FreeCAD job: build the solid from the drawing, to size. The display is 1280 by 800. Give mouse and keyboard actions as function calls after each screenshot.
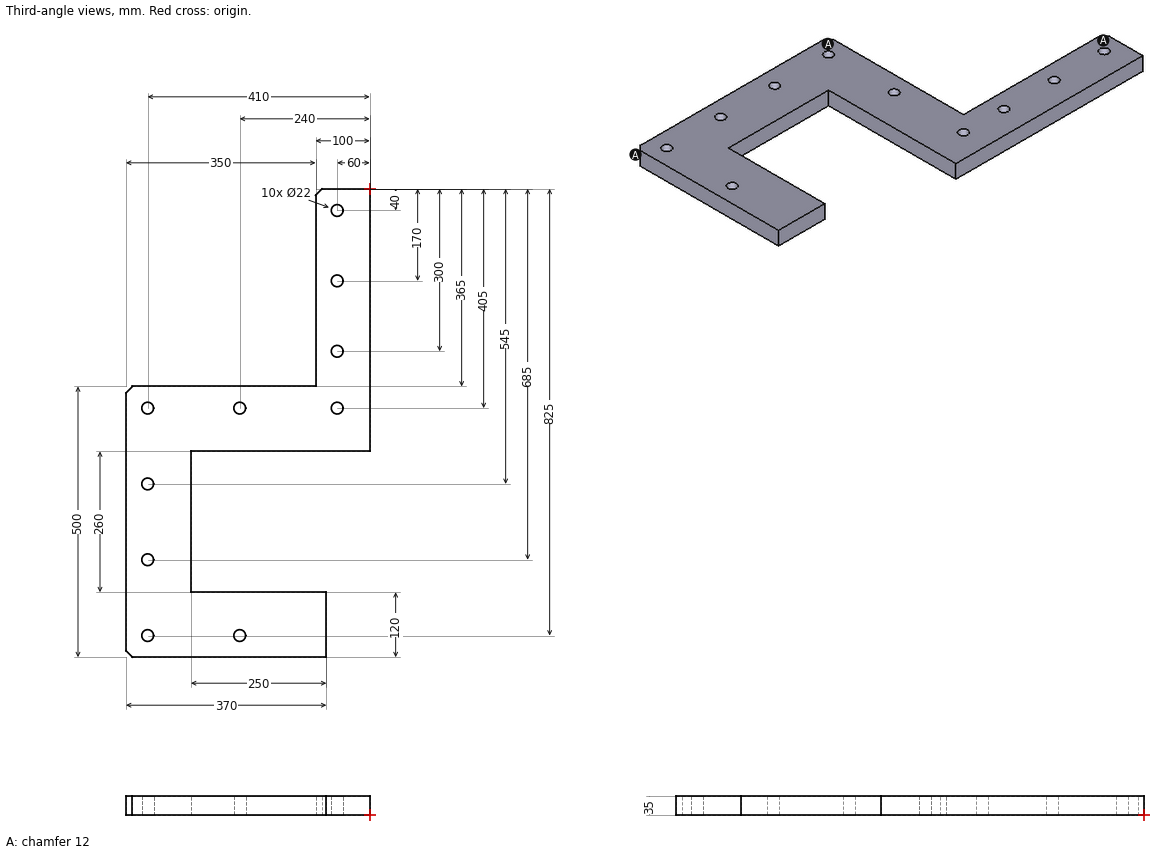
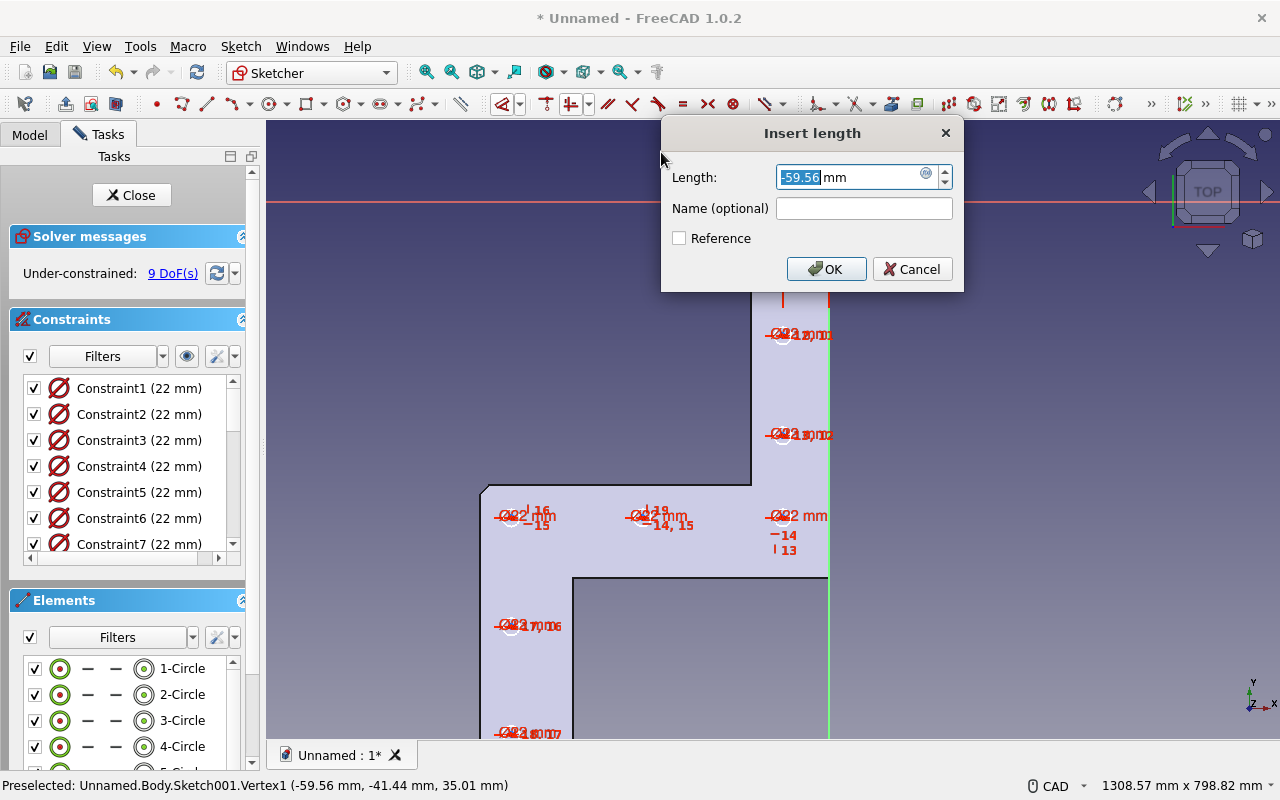
text(-60)
key(Return)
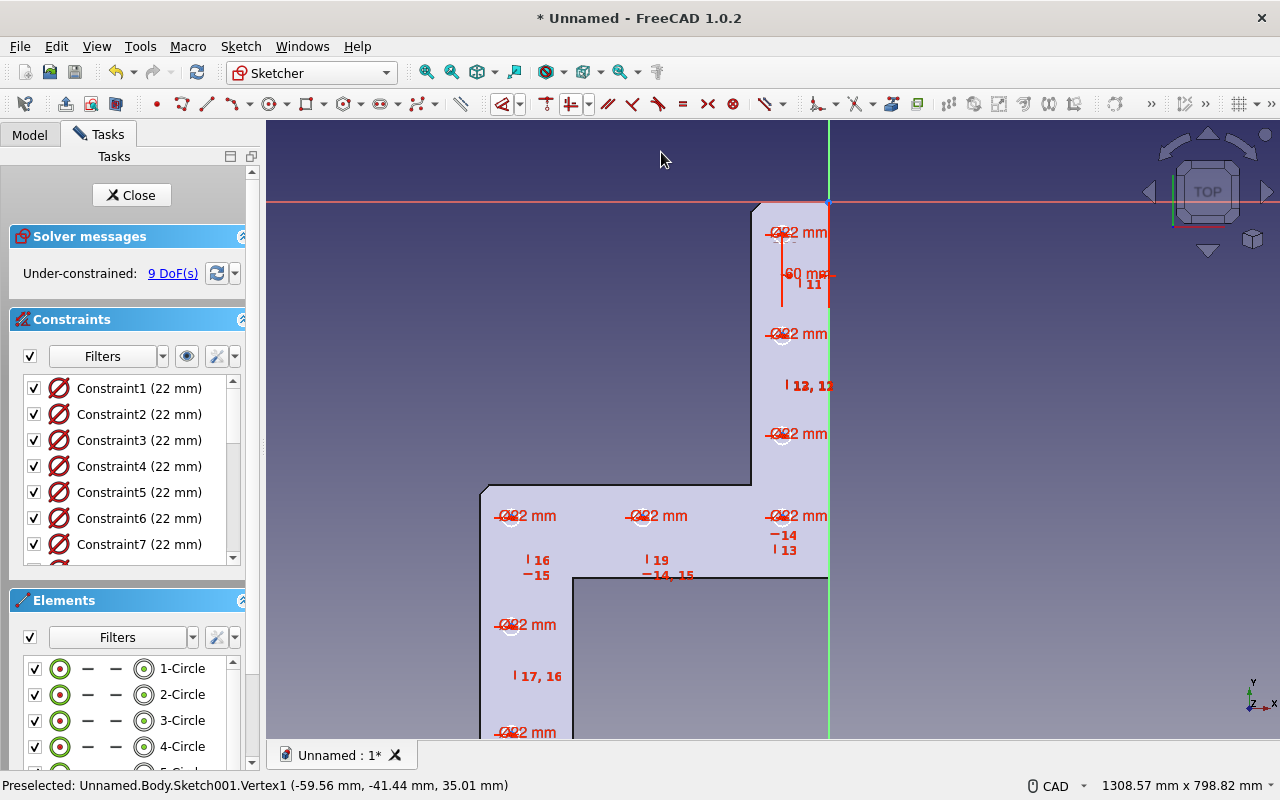
scroll(782, 235, up, 2)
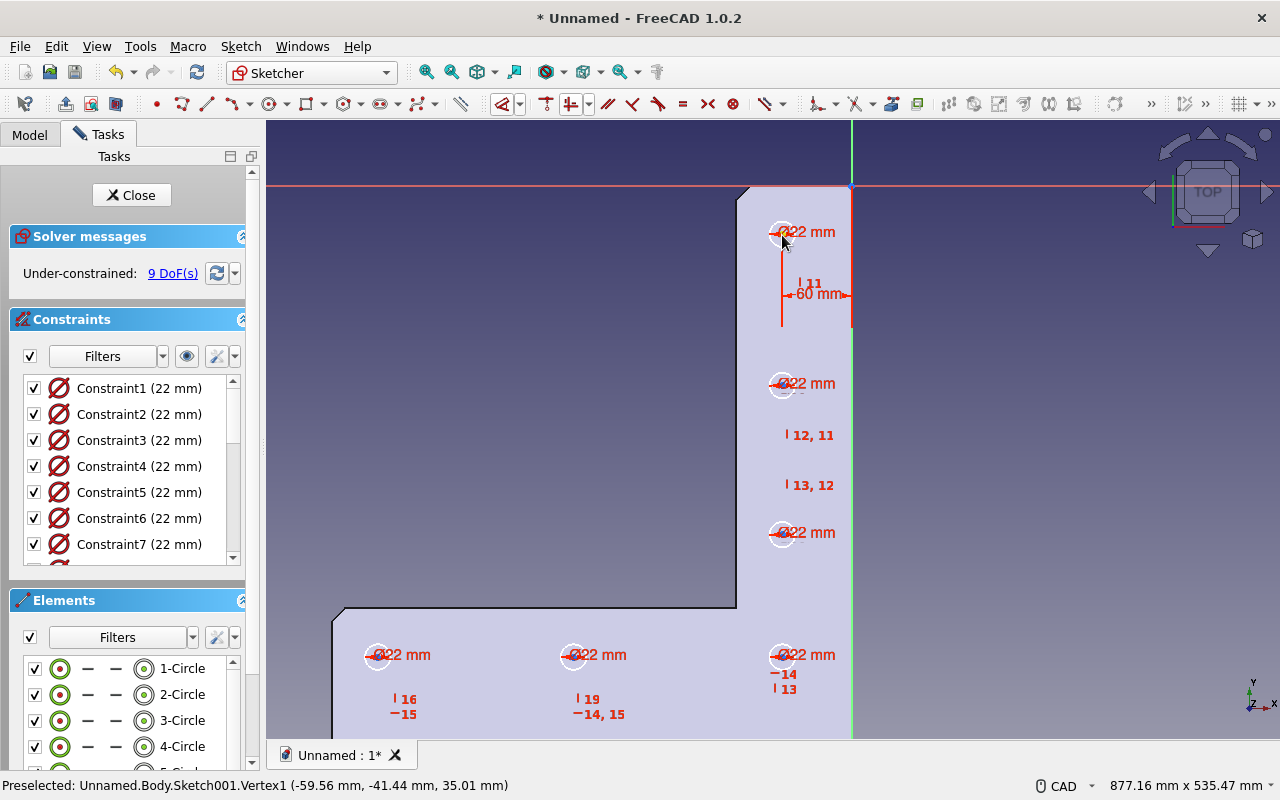
click(782, 234)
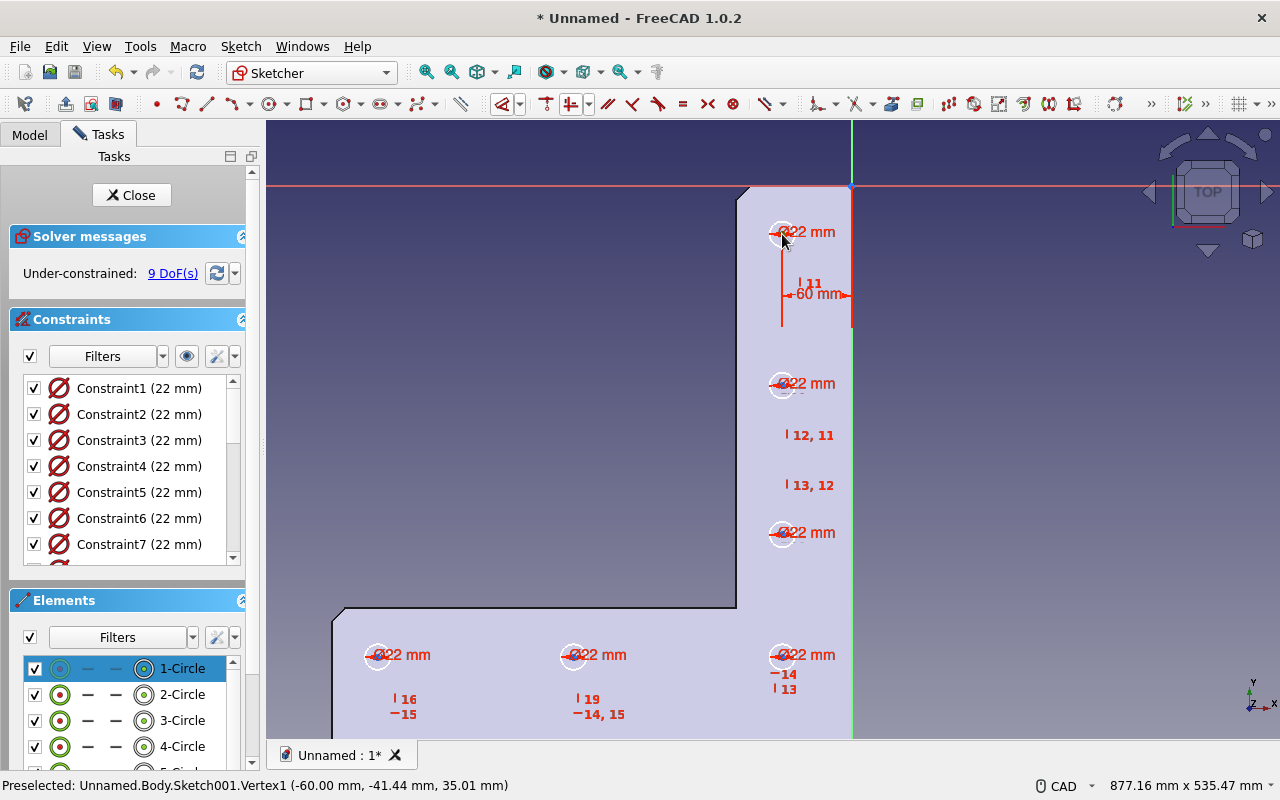
click(520, 104)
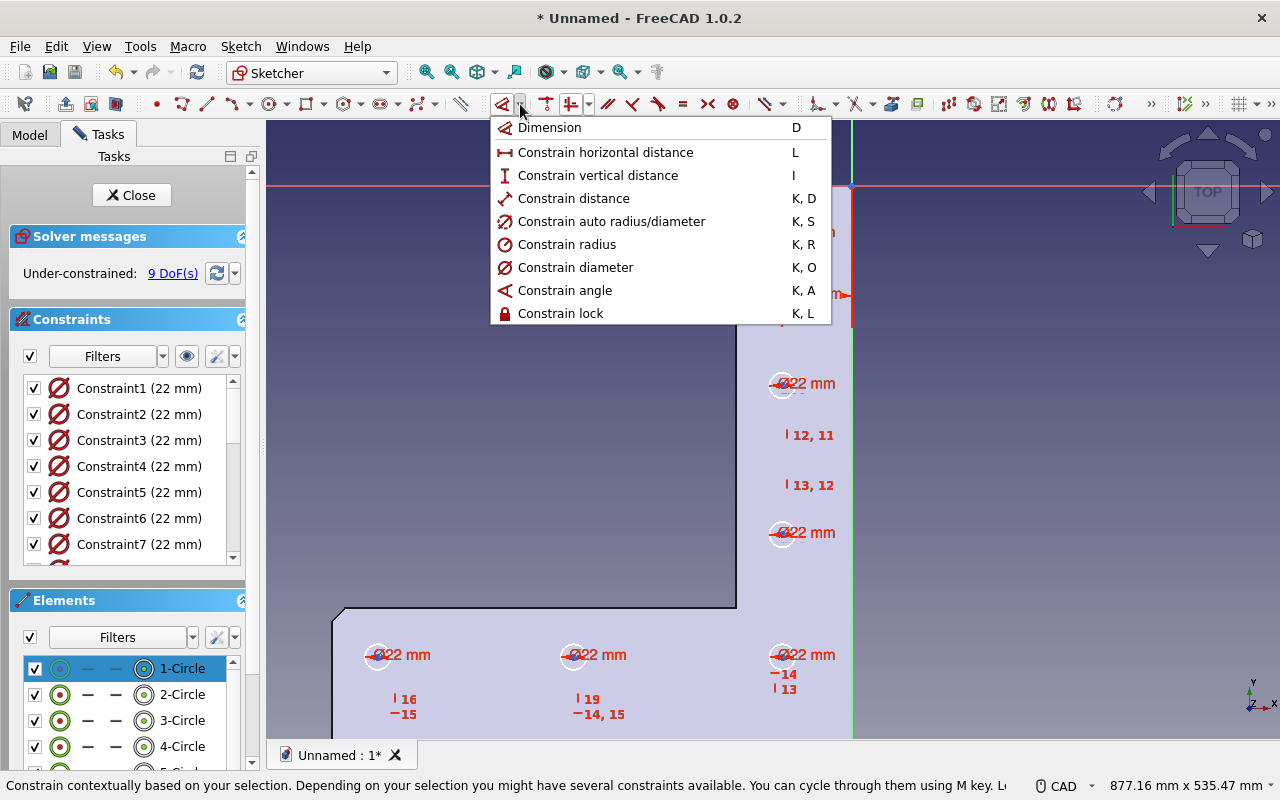
click(661, 176)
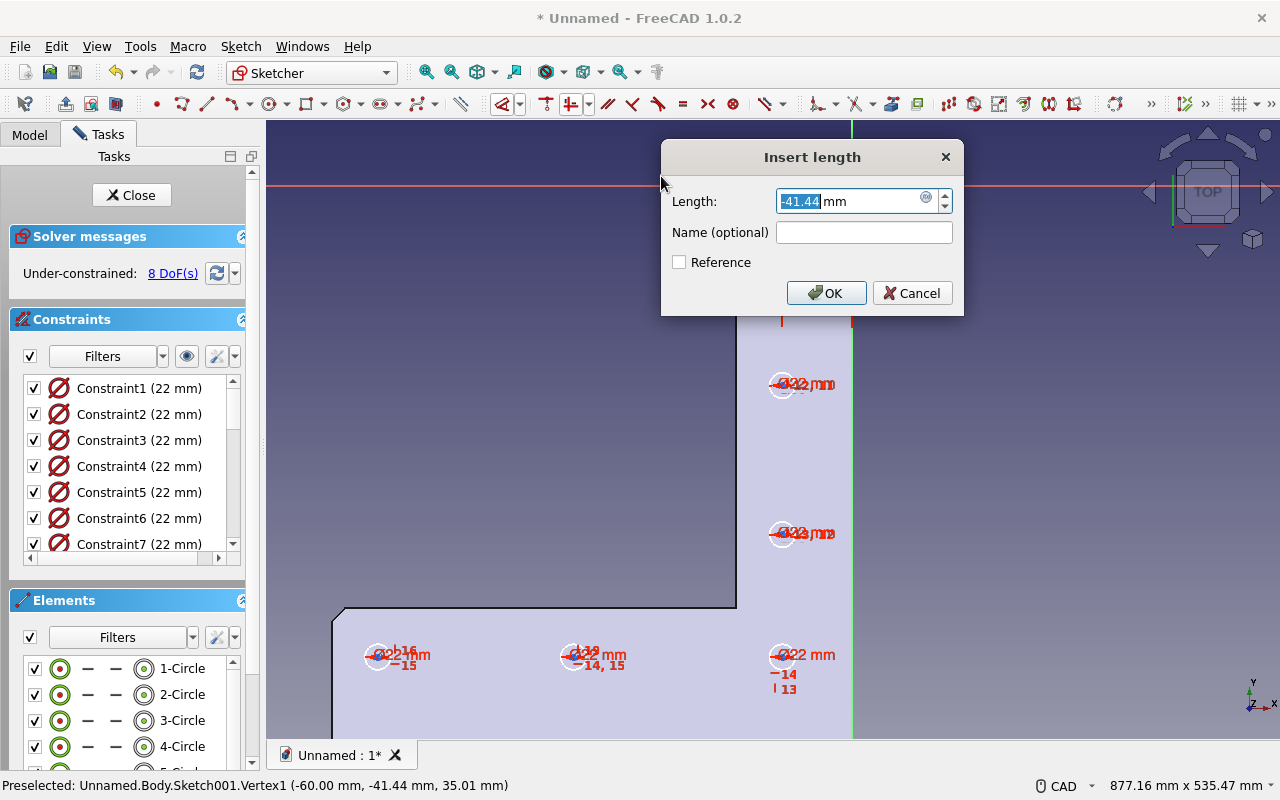
text(-40)
key(Return)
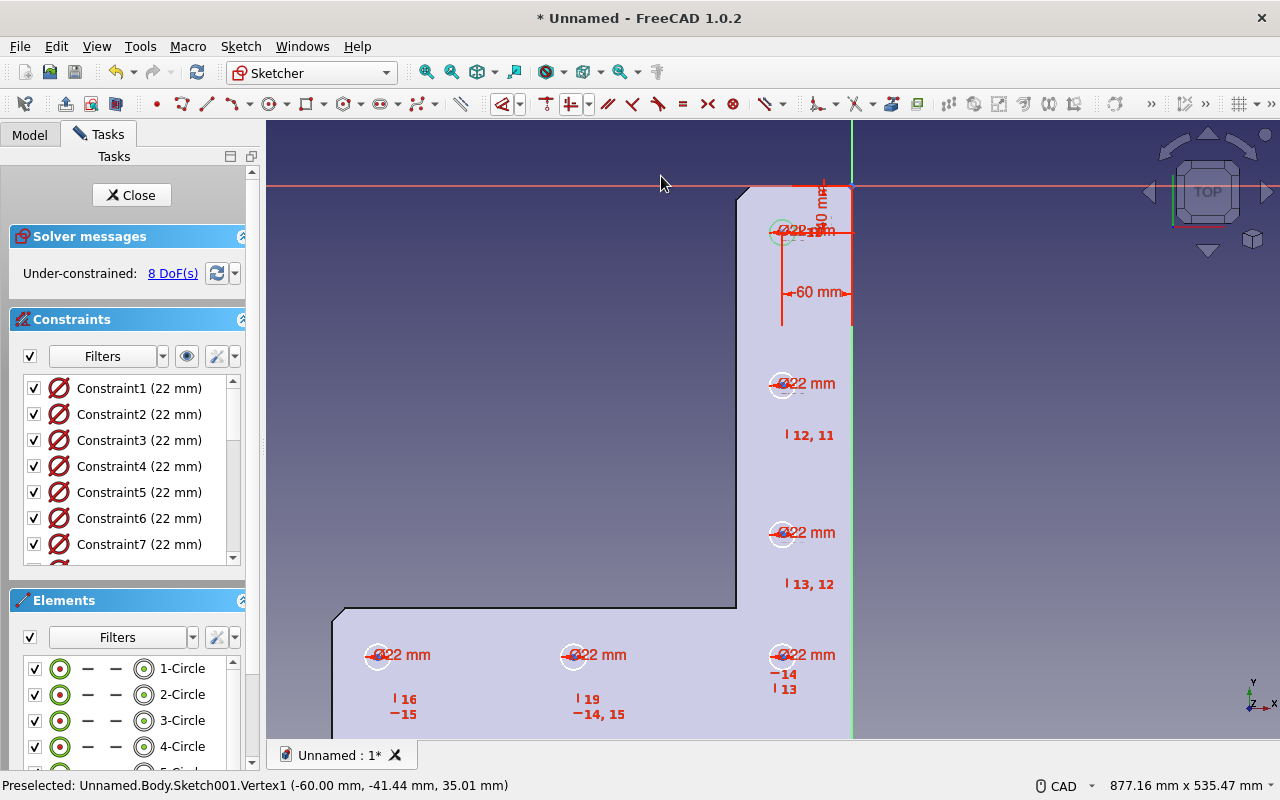
click(782, 386)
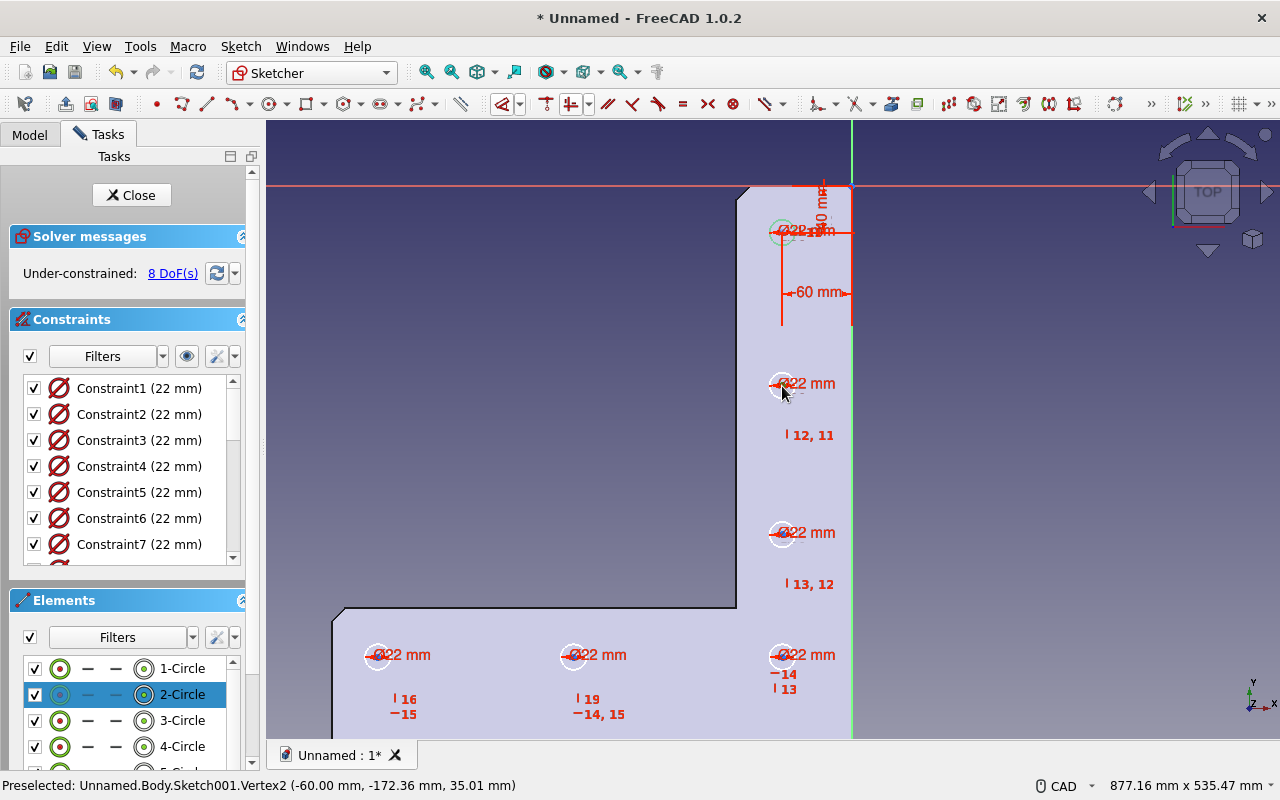
click(520, 104)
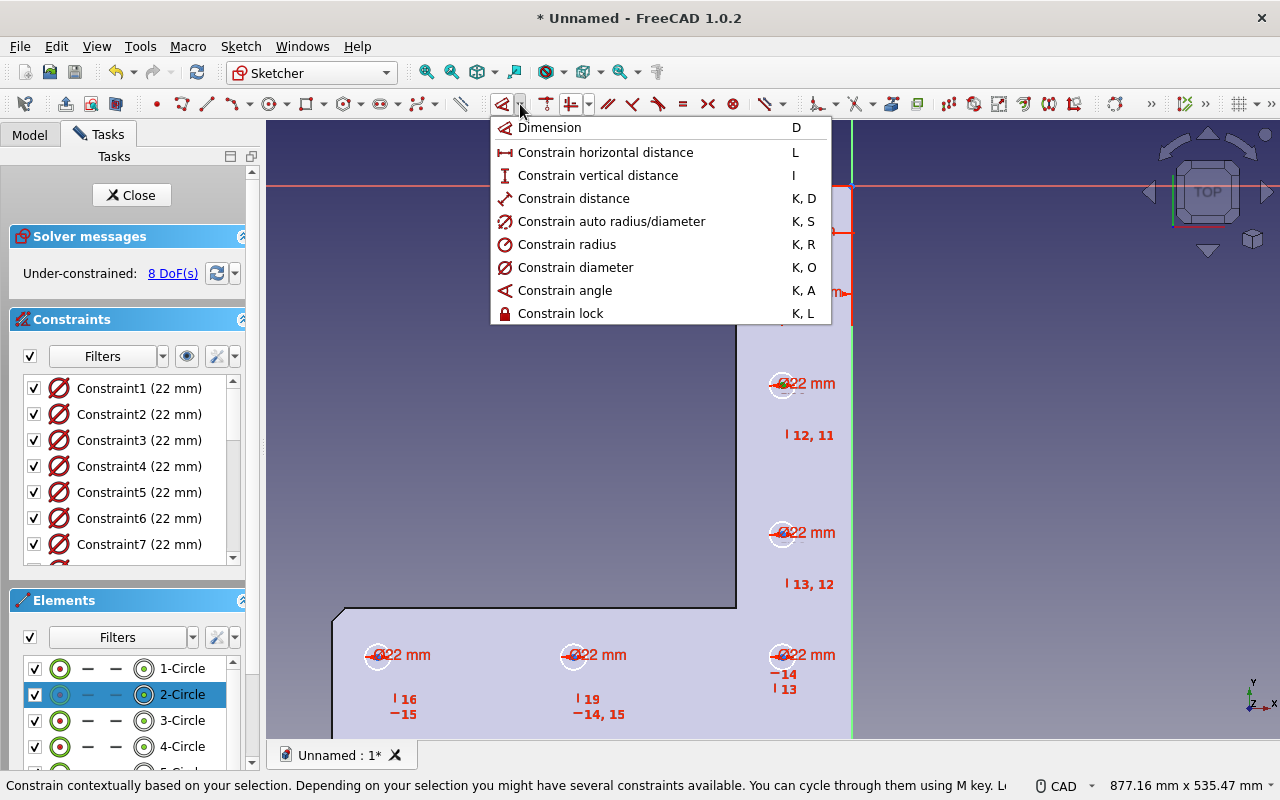
click(661, 176)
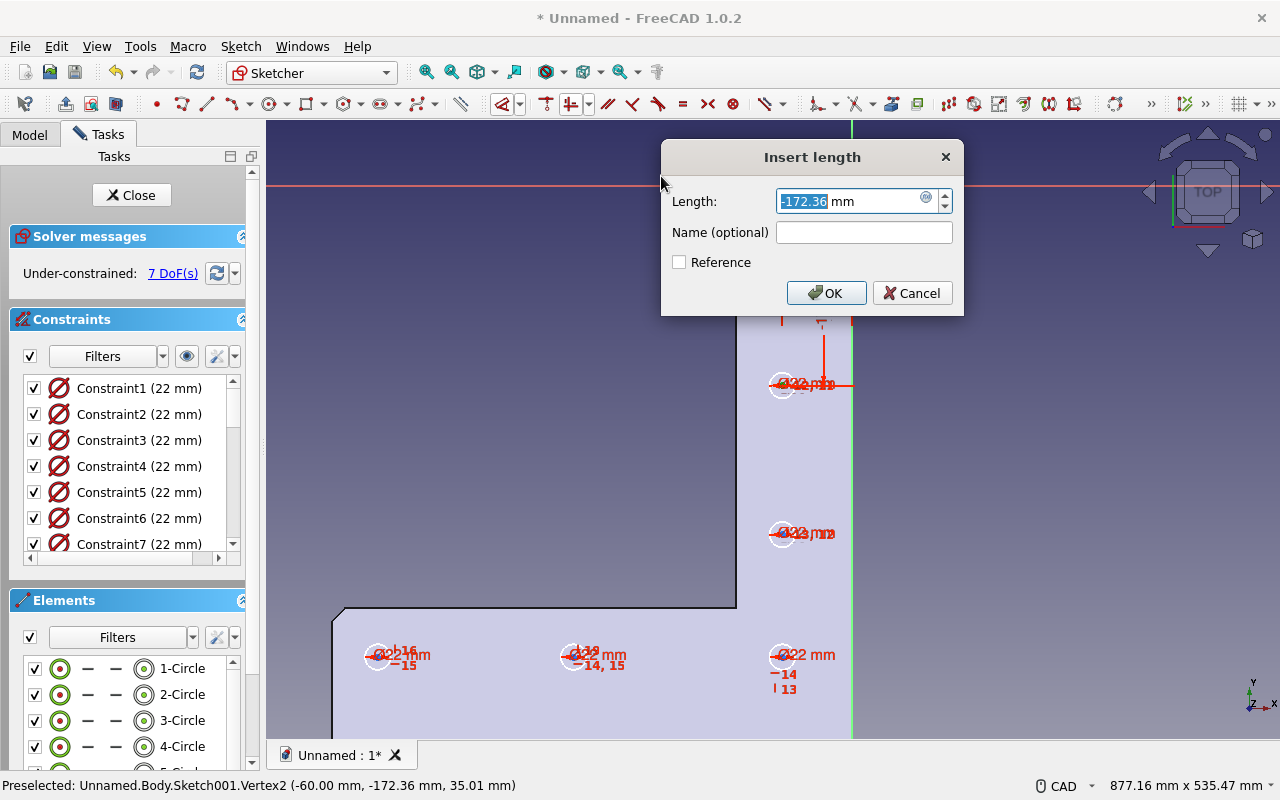
text(-170)
key(Return)